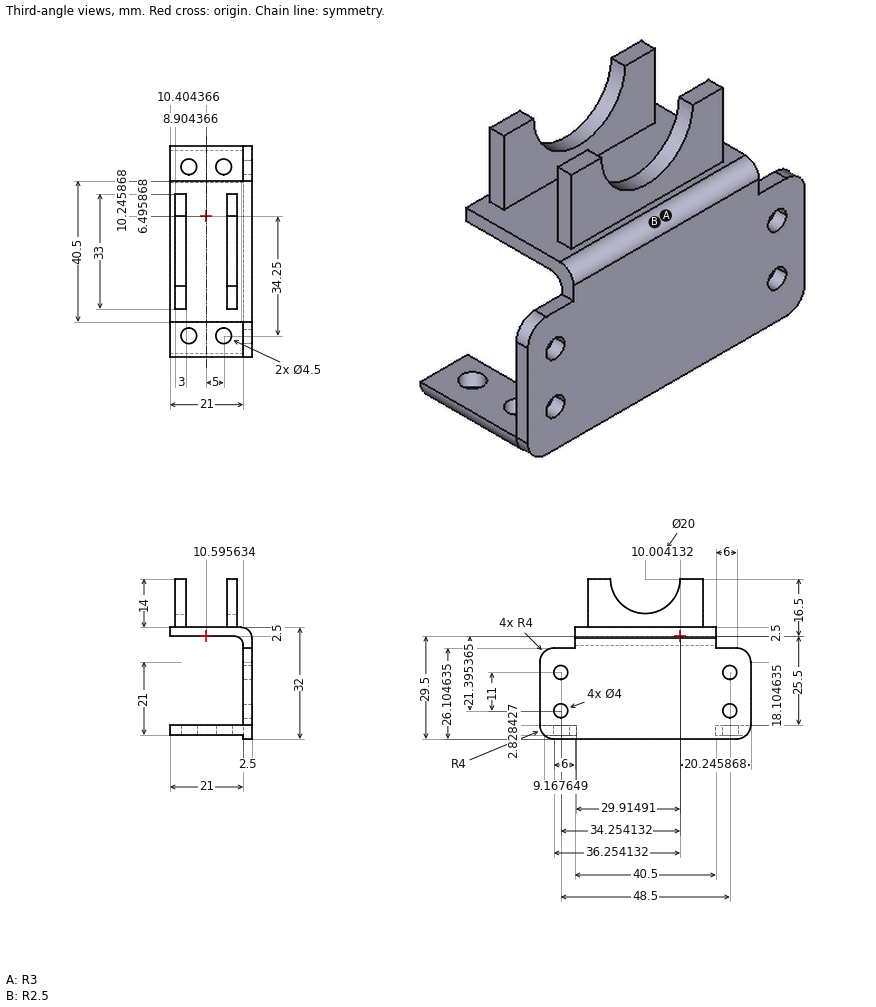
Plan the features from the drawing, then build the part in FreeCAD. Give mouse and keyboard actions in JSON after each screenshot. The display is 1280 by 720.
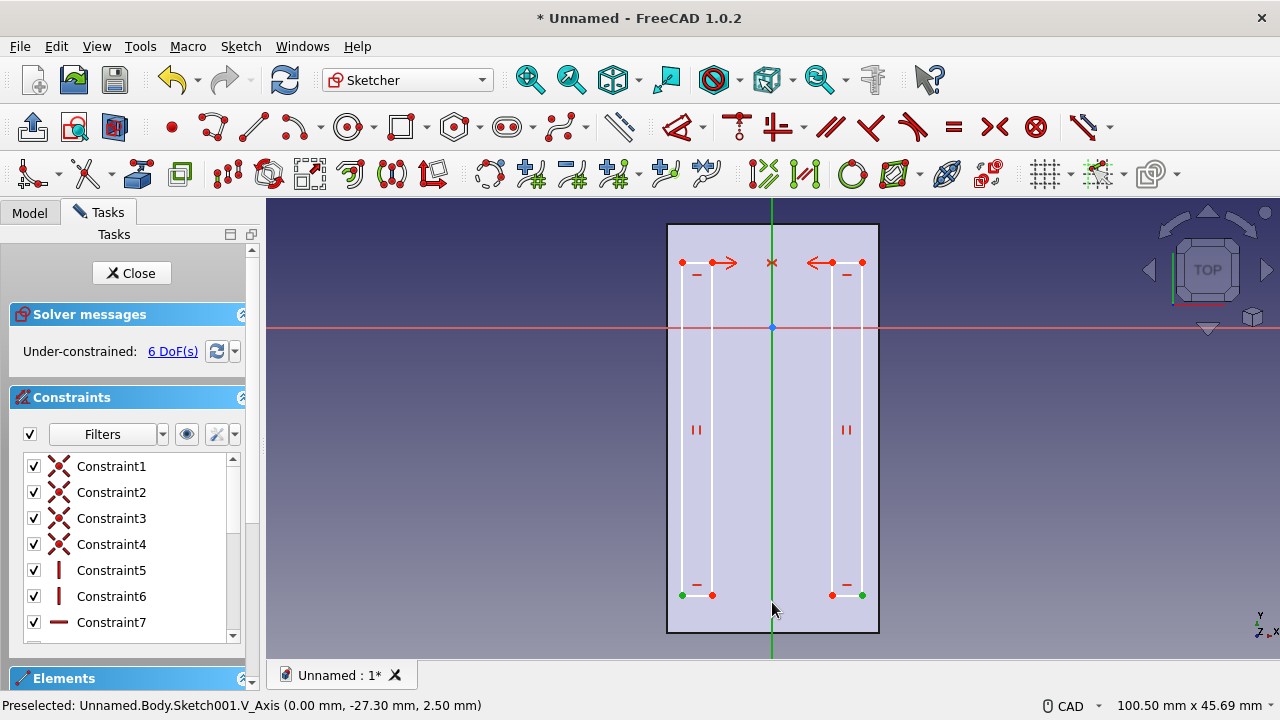
{"action": "left_click", "coordinate": [995, 128]}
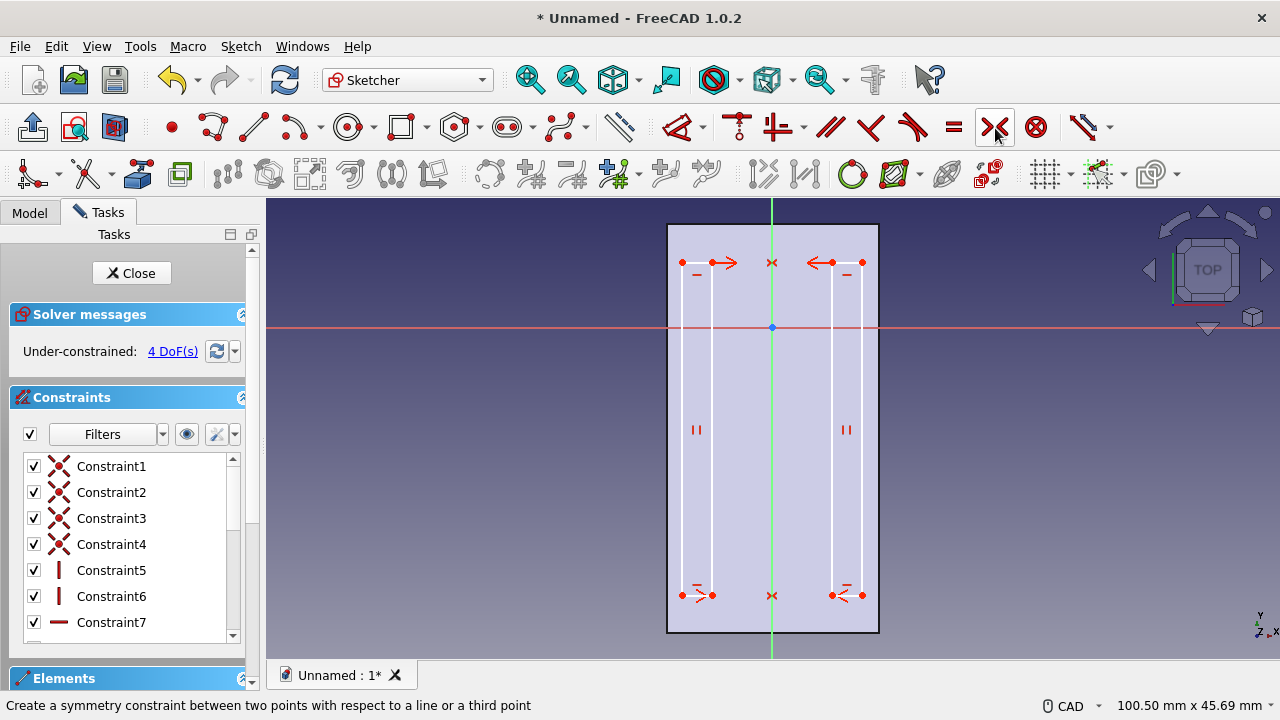
{"action": "left_click", "coordinate": [676, 128]}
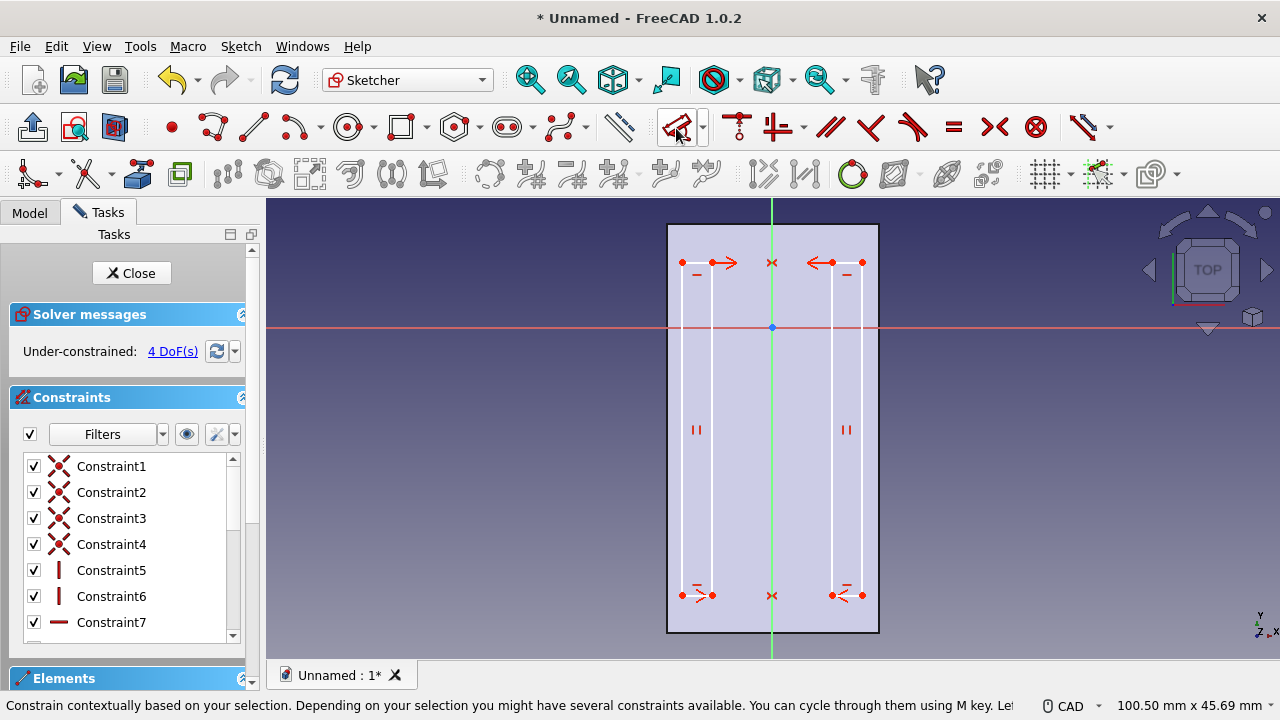
{"action": "scroll", "coordinate": [694, 596], "scroll_direction": "up", "scroll_amount": 2}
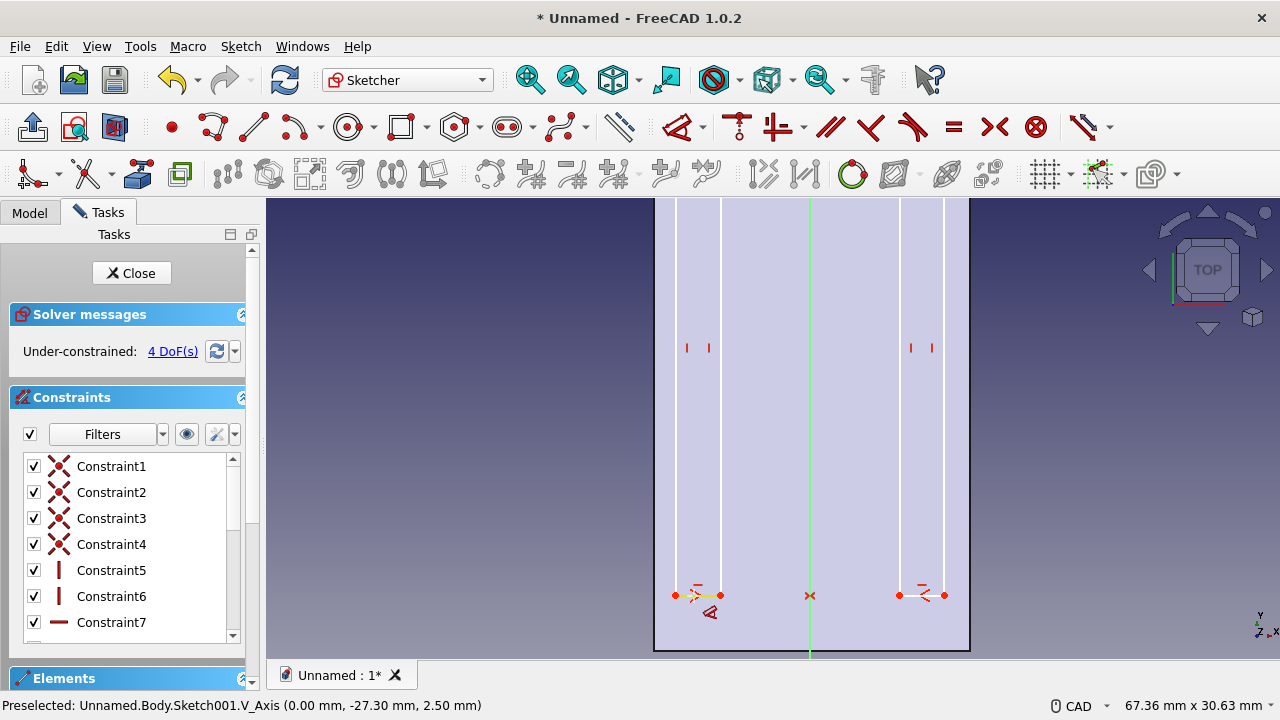
{"action": "left_click", "coordinate": [694, 596]}
{"action": "left_click", "coordinate": [698, 630]}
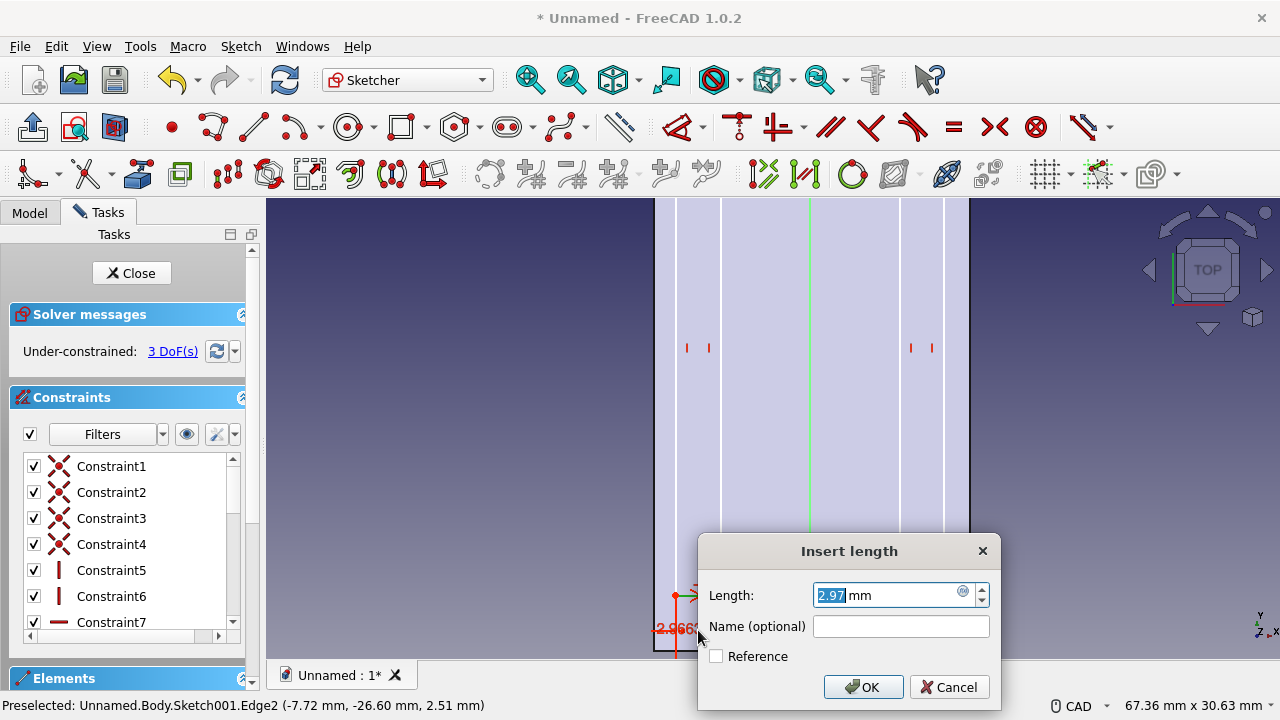
{"action": "type", "text": "3"}
{"action": "key", "text": "Return"}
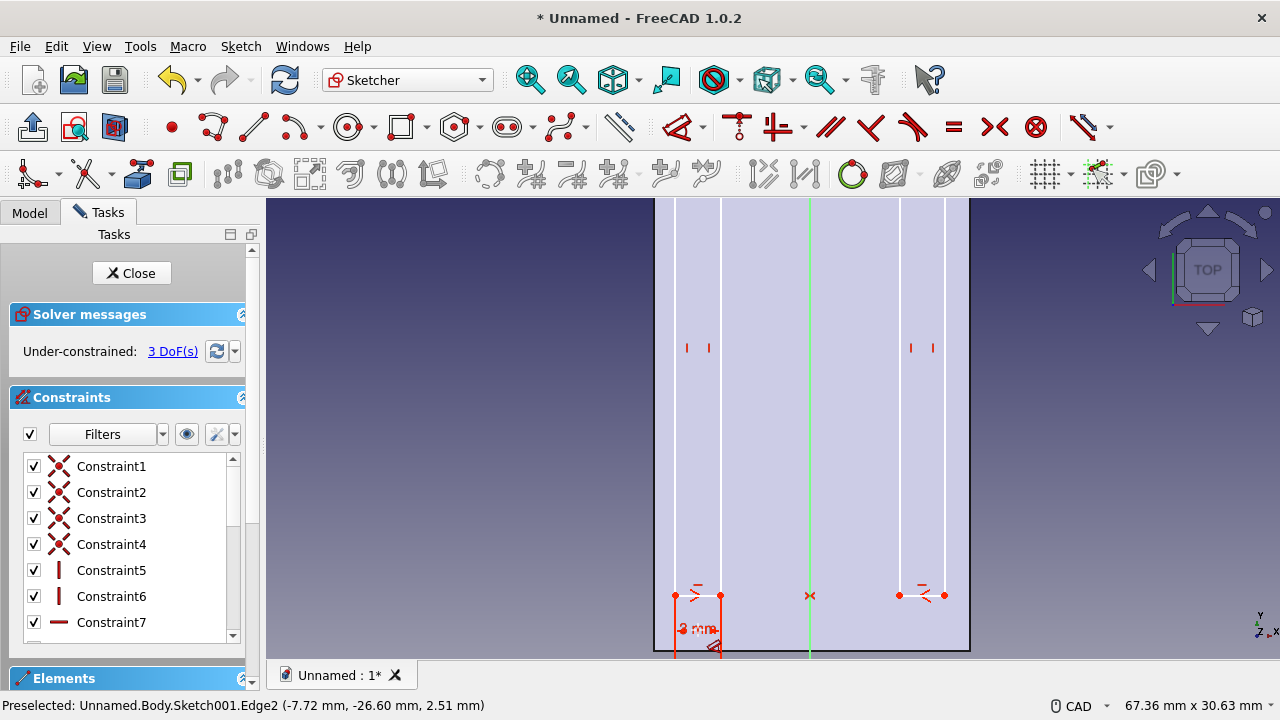
{"action": "left_click", "coordinate": [675, 248]}
{"action": "left_click", "coordinate": [641, 411]}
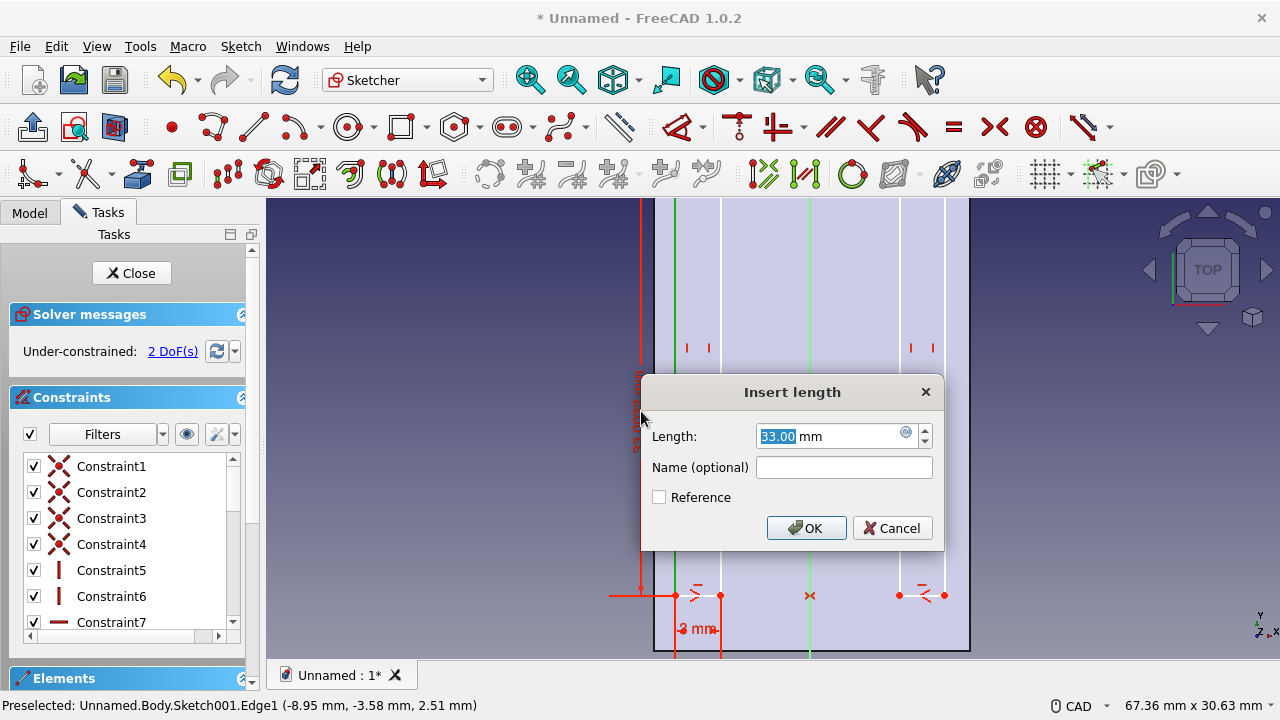
{"action": "type", "text": "33"}
{"action": "key", "text": "Return"}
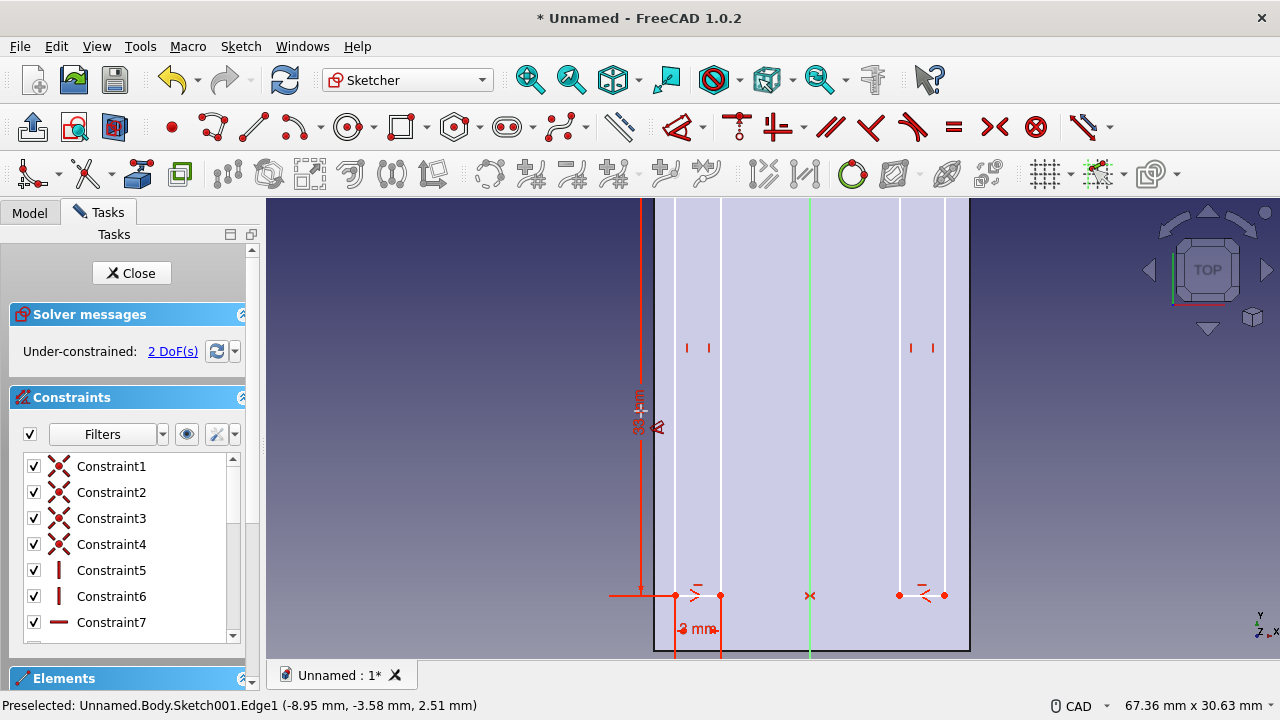
{"action": "scroll", "coordinate": [576, 529], "scroll_direction": "down", "scroll_amount": 3}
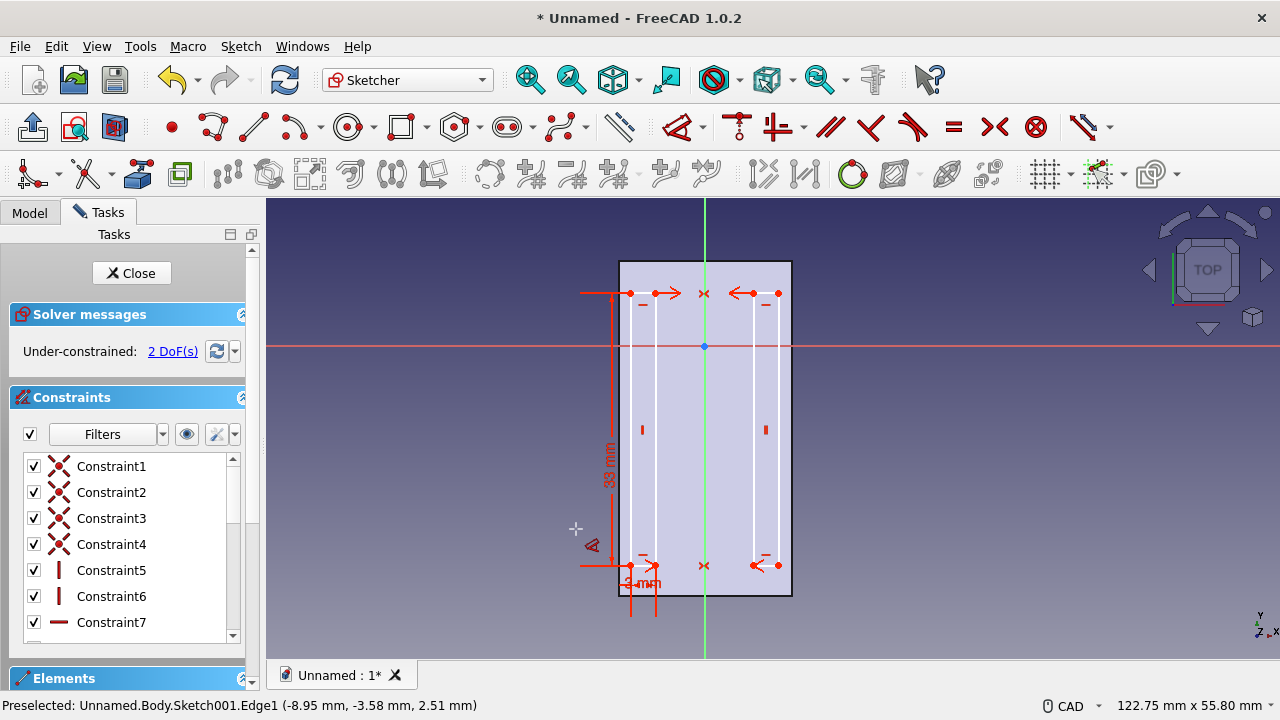
{"action": "left_click", "coordinate": [631, 293]}
{"action": "left_click", "coordinate": [668, 259]}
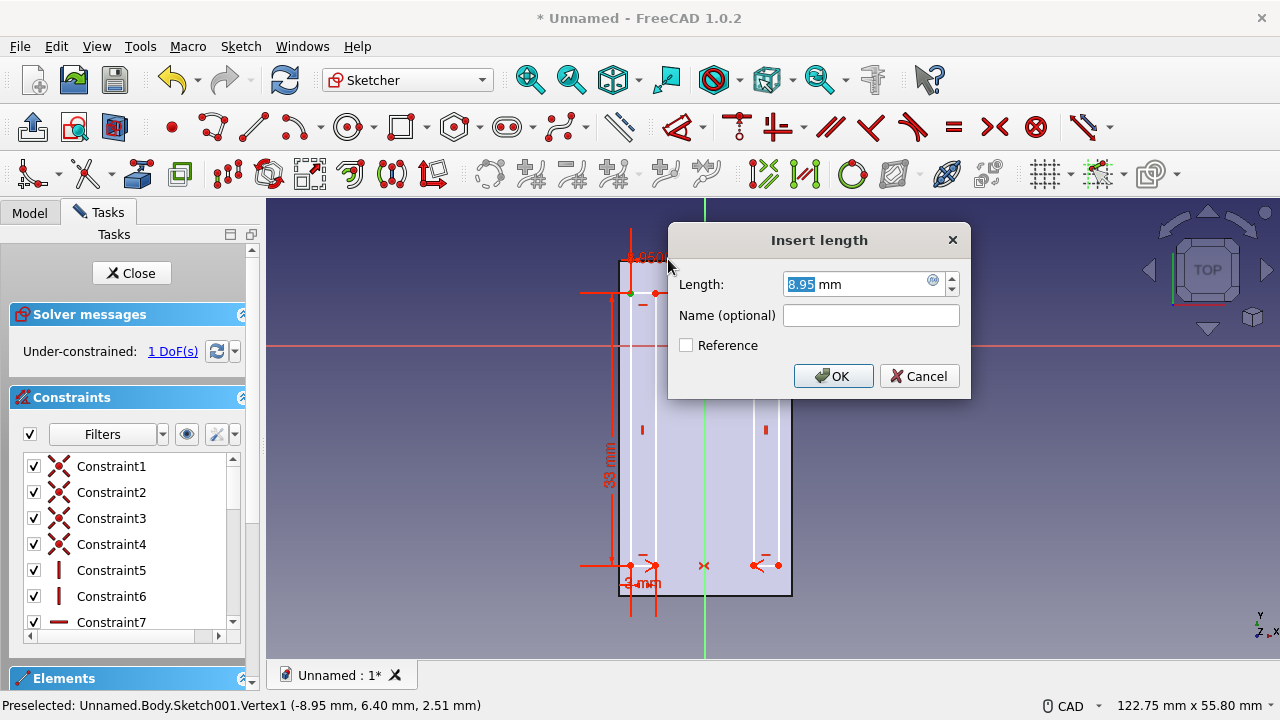
{"action": "type", "text": "8.904366"}
{"action": "key", "text": "Return"}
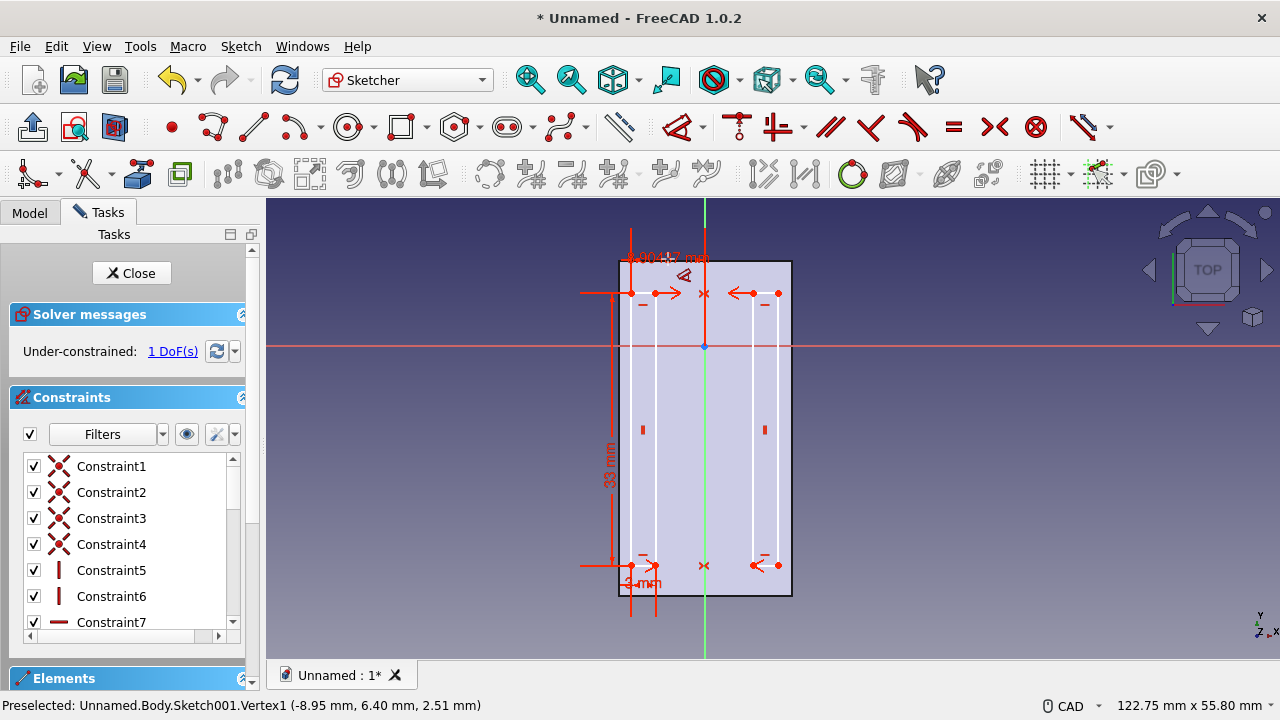
{"action": "left_click", "coordinate": [631, 293]}
{"action": "left_click", "coordinate": [597, 320]}